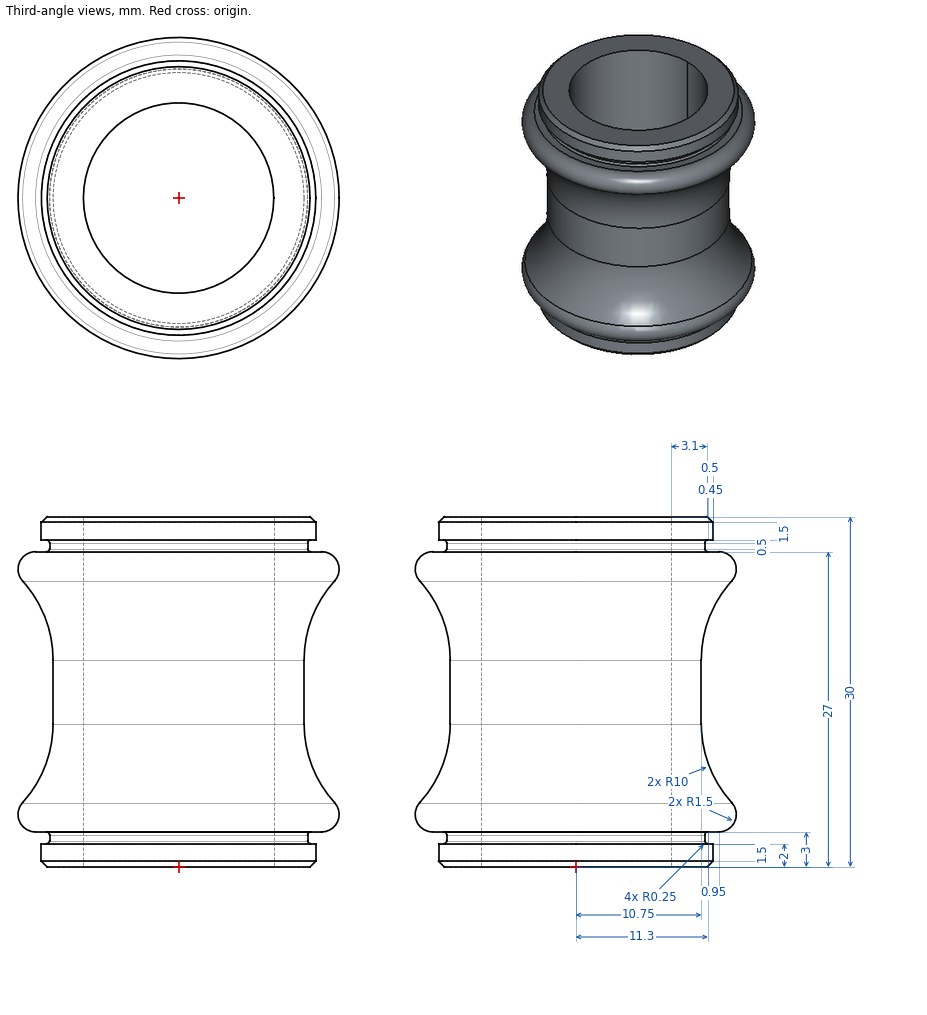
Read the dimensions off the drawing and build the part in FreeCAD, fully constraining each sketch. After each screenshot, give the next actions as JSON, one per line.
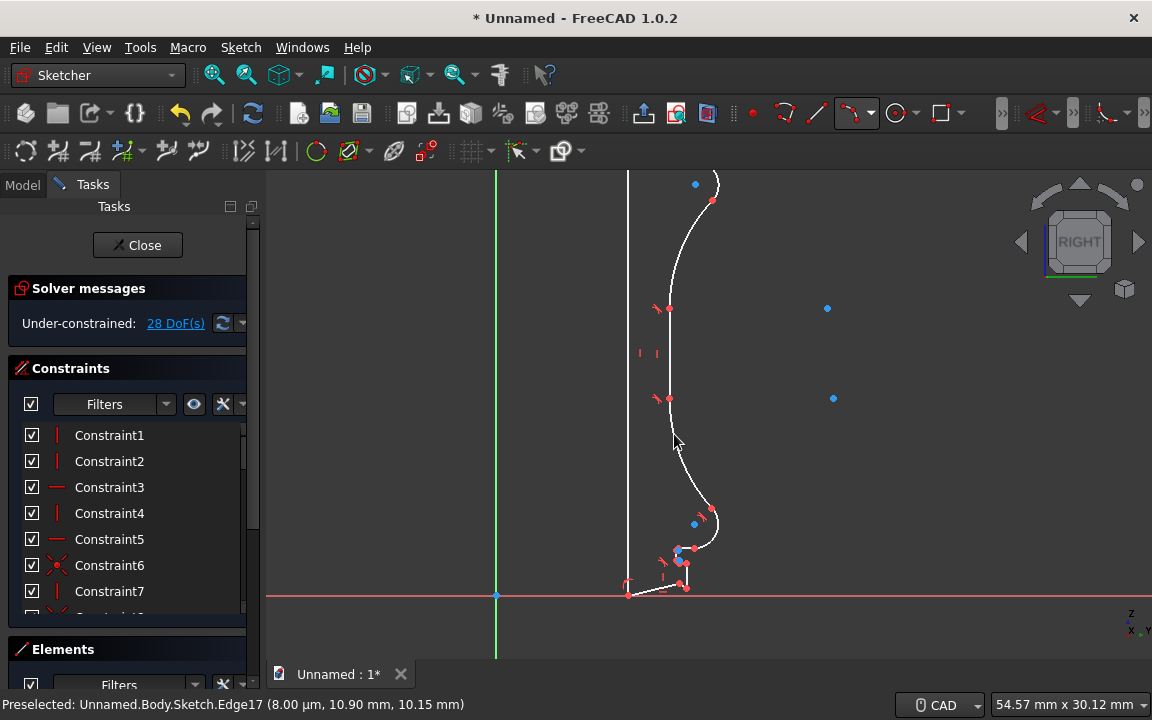
{"action": "left_click", "coordinate": [691, 229]}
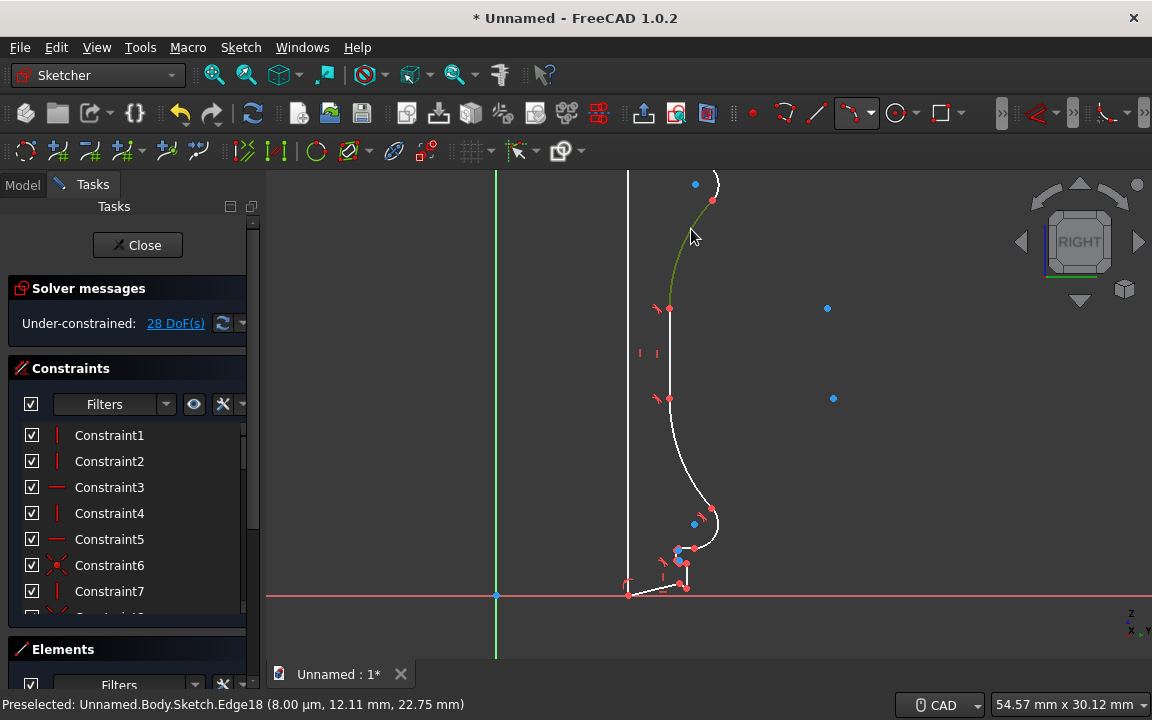
{"action": "scroll", "coordinate": [709, 541], "scroll_direction": "down", "scroll_amount": 2}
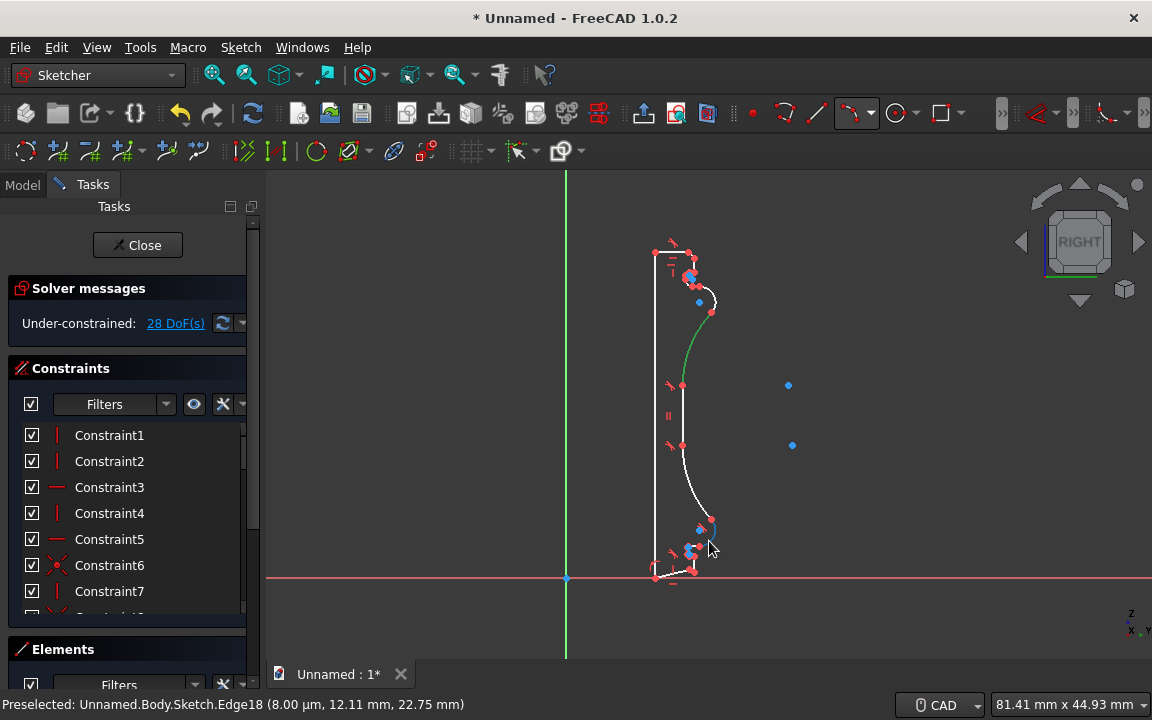
{"action": "scroll", "coordinate": [716, 303], "scroll_direction": "up", "scroll_amount": 2}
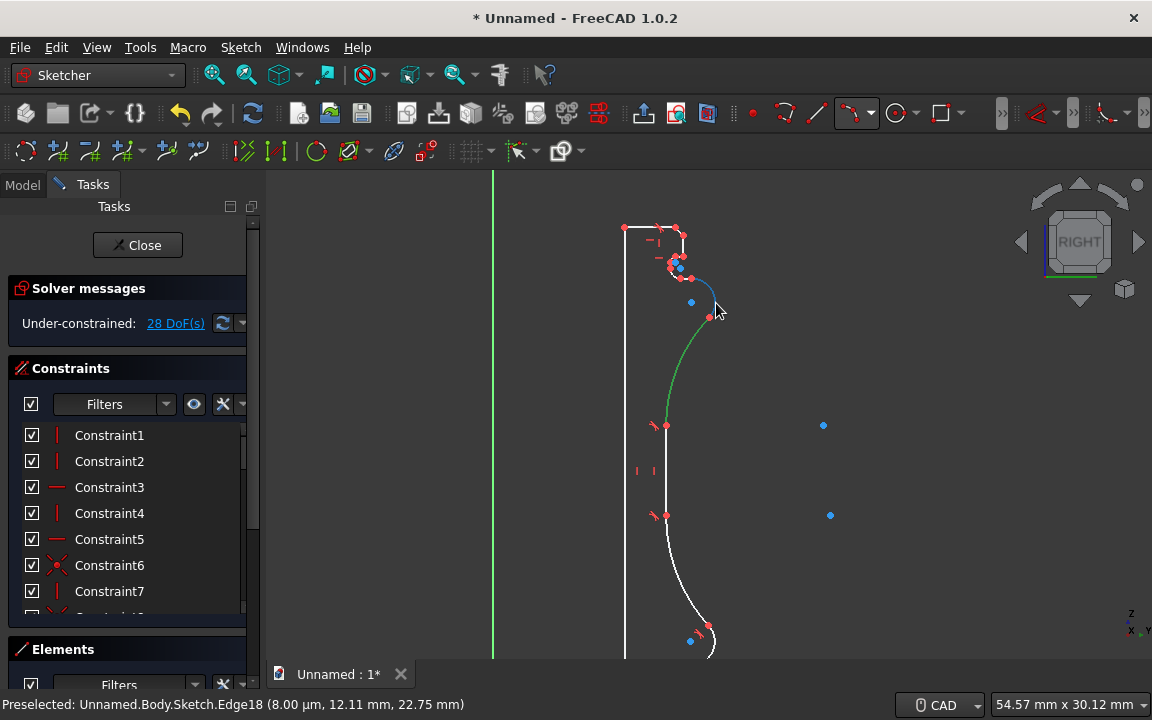
{"action": "left_click", "coordinate": [715, 303]}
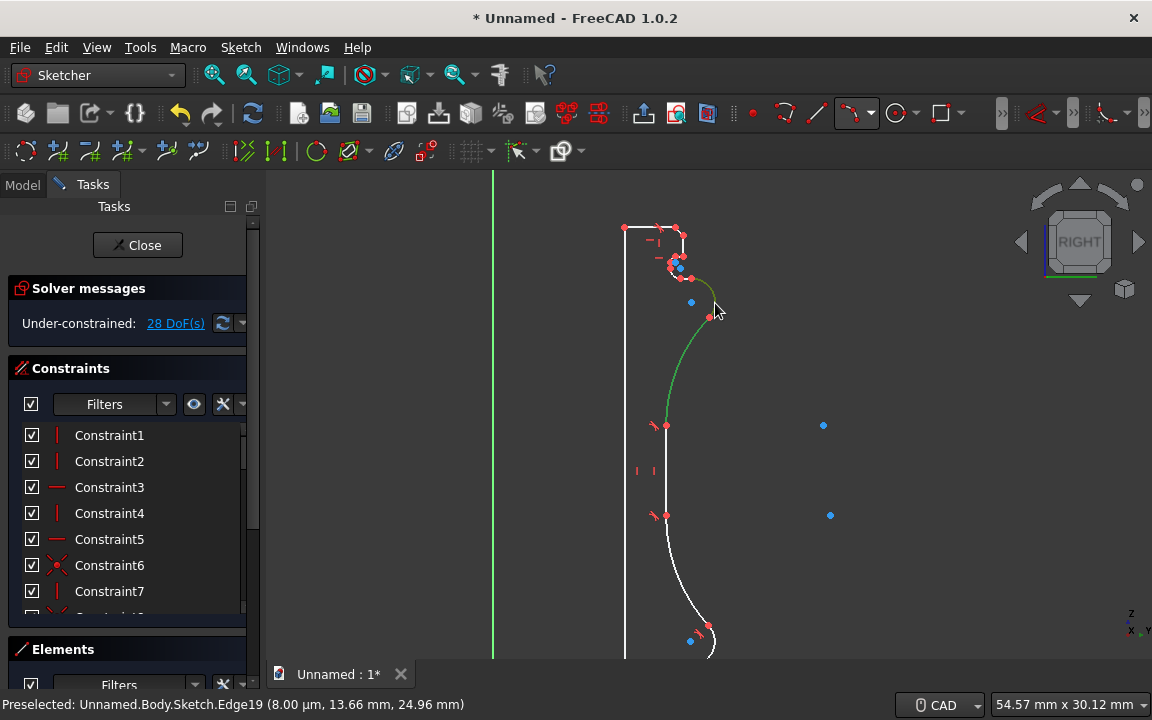
{"action": "key", "text": "t"}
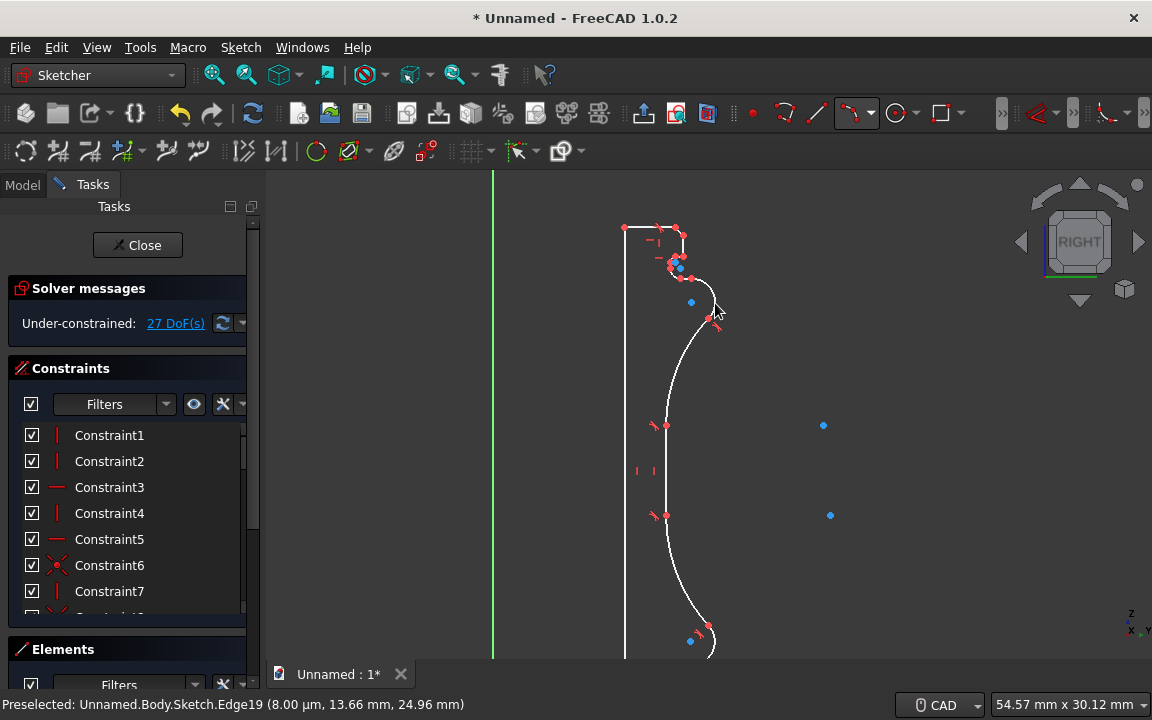
{"action": "scroll", "coordinate": [716, 302], "scroll_direction": "down", "scroll_amount": 2}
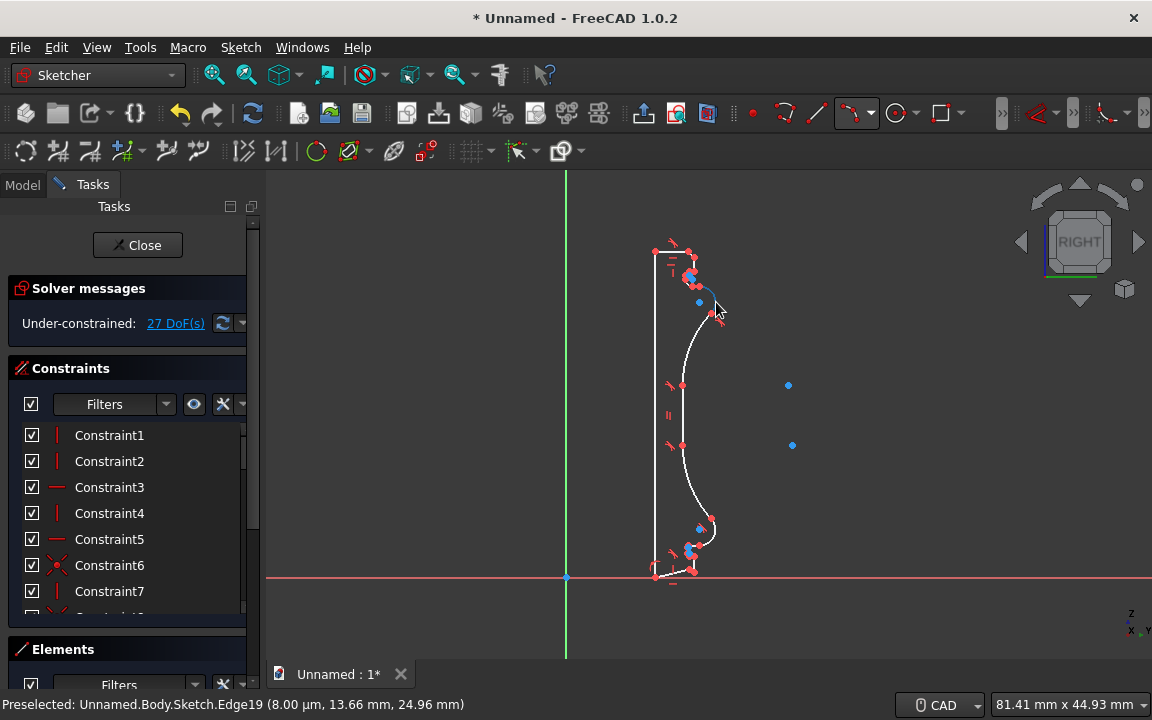
{"action": "scroll", "coordinate": [694, 546], "scroll_direction": "up", "scroll_amount": 5}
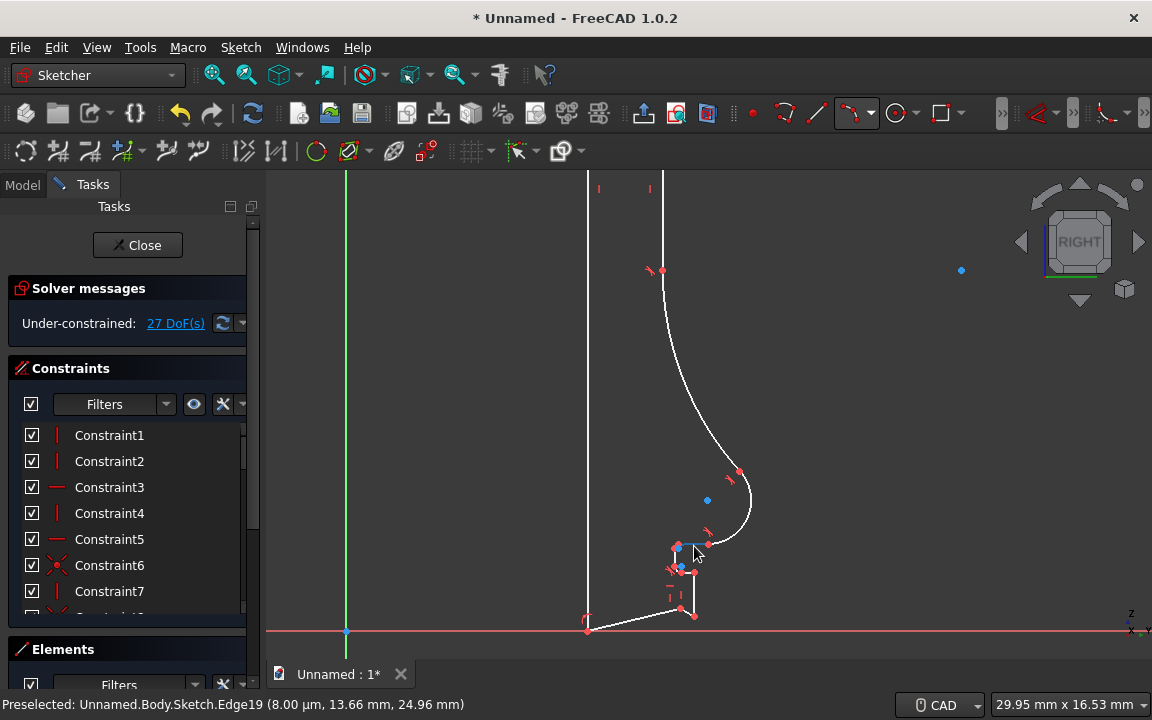
{"action": "left_click", "coordinate": [694, 544]}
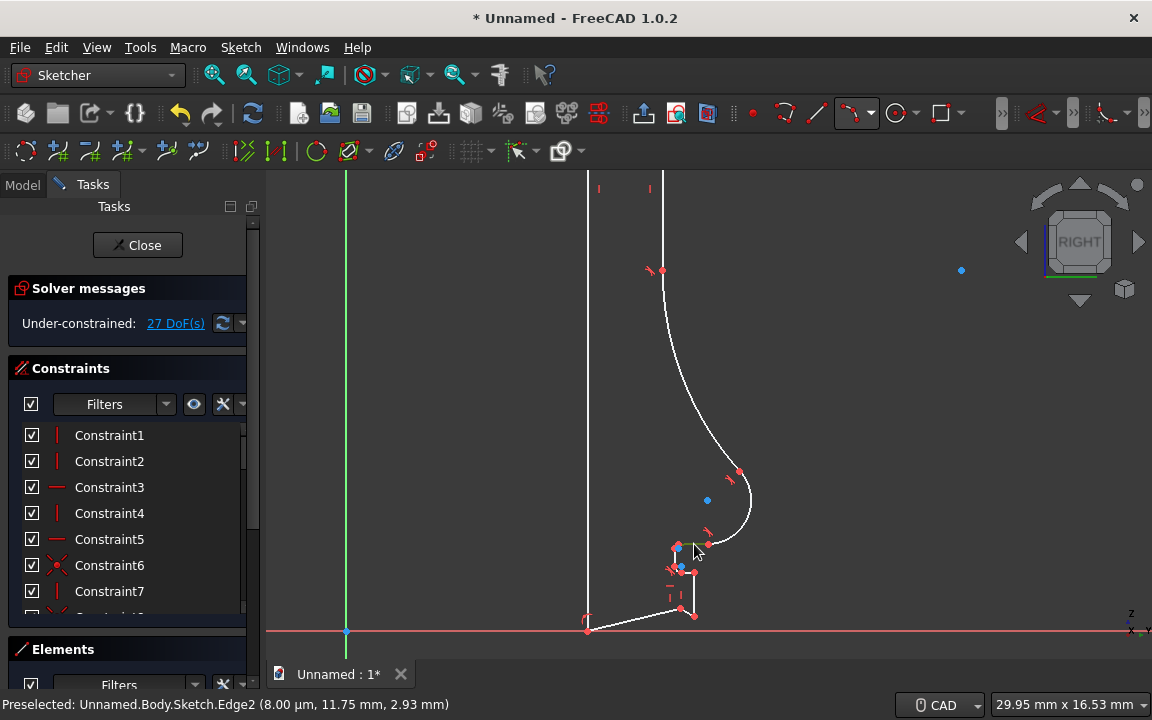
{"action": "key", "text": "h"}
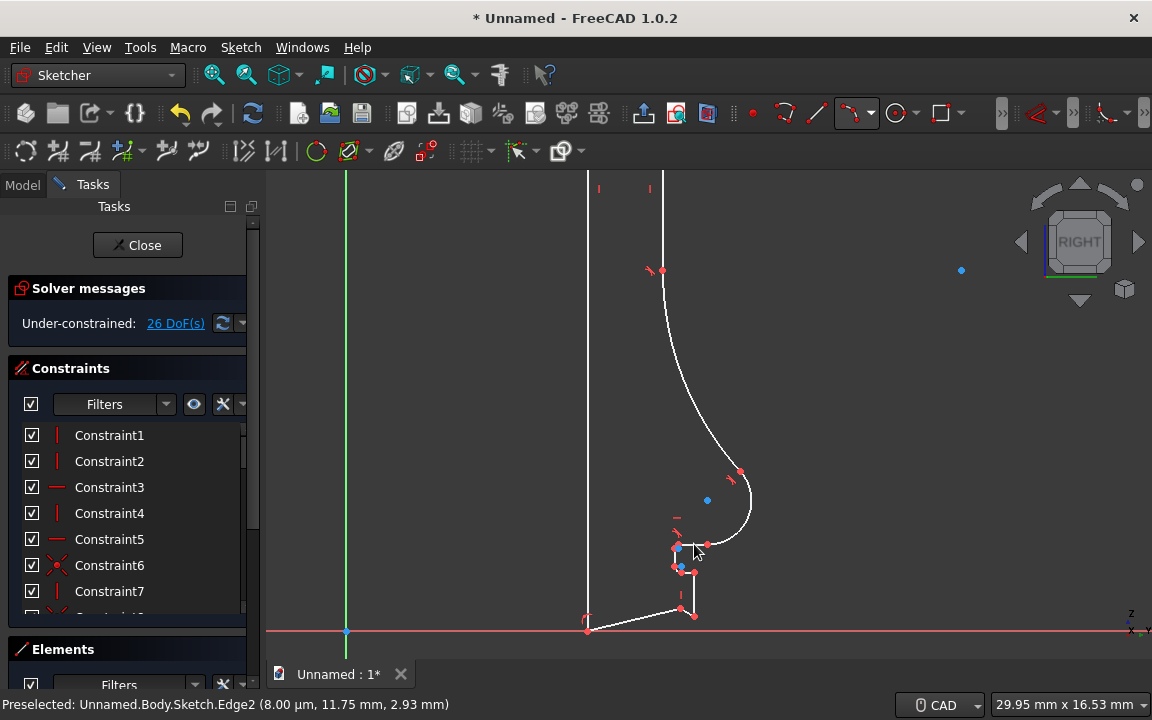
{"action": "left_click", "coordinate": [653, 615]}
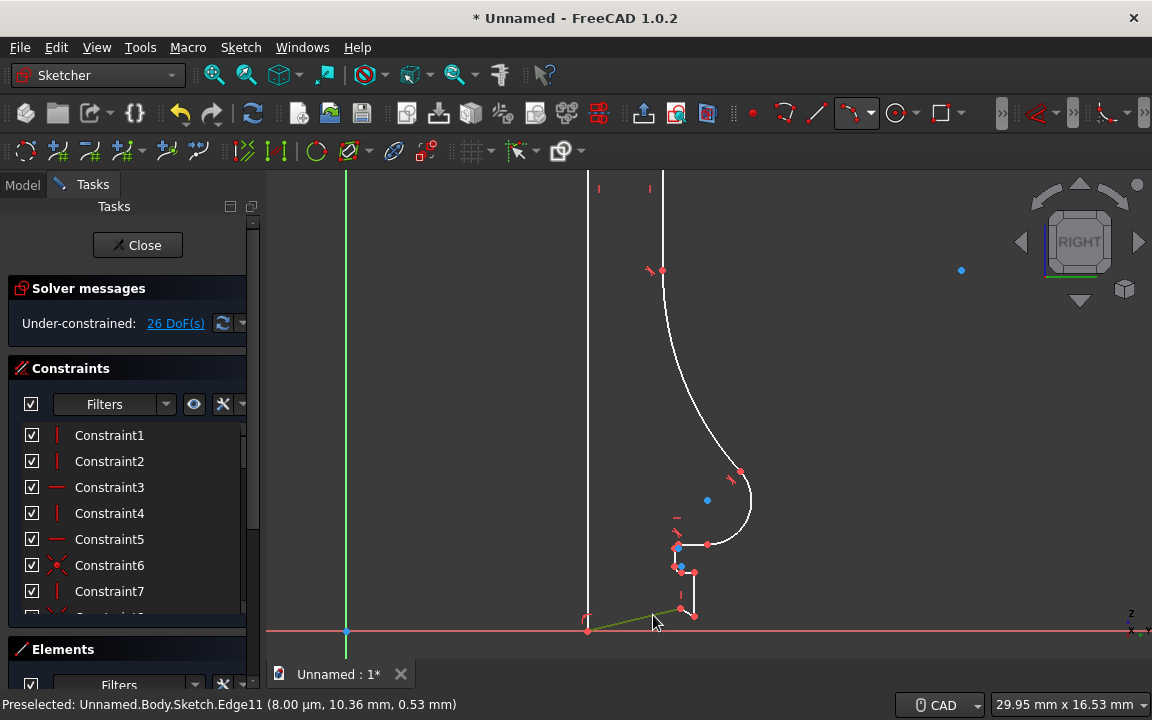
{"action": "key", "text": "h"}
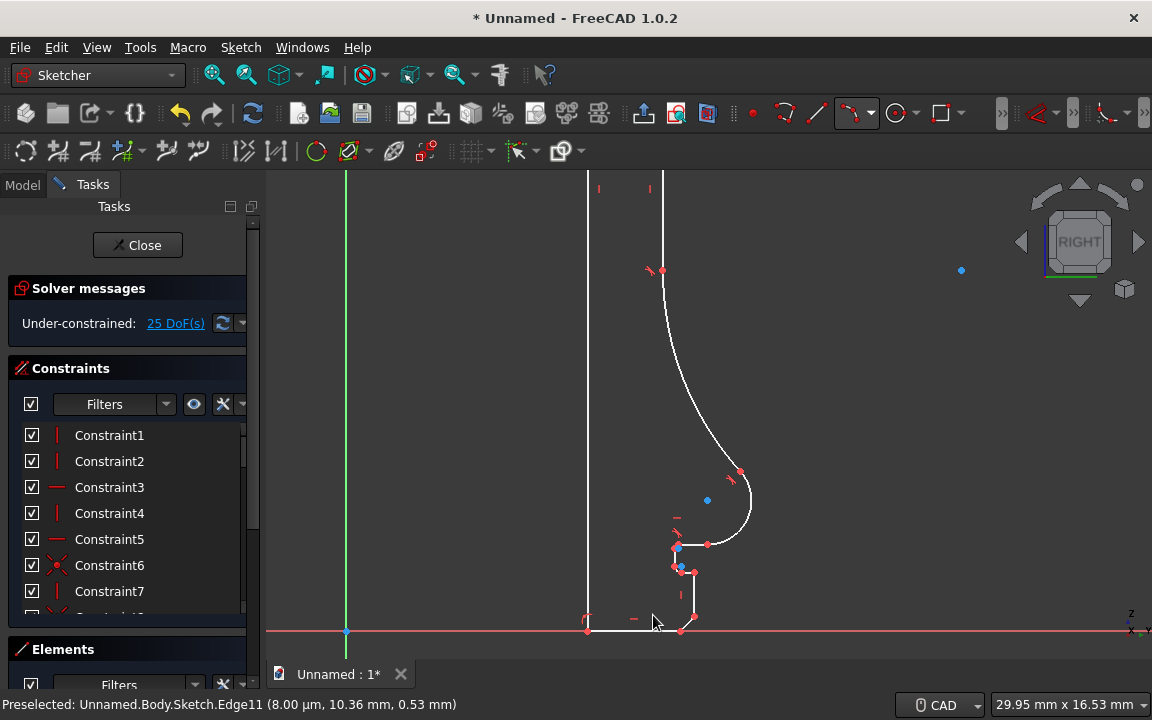
{"action": "left_click", "coordinate": [670, 336]}